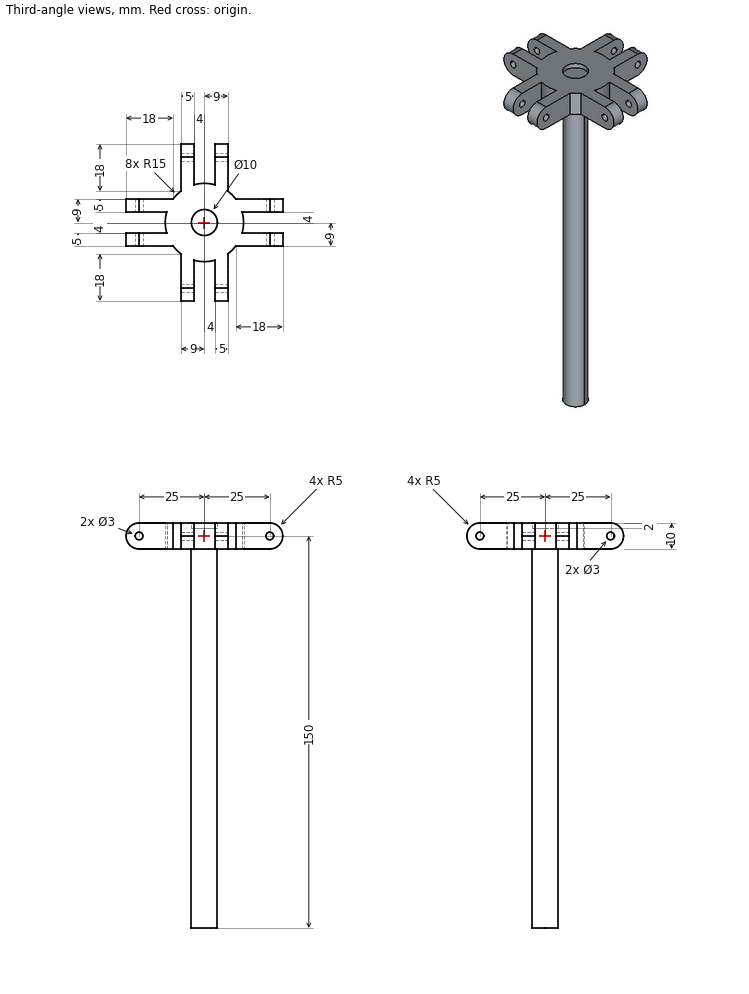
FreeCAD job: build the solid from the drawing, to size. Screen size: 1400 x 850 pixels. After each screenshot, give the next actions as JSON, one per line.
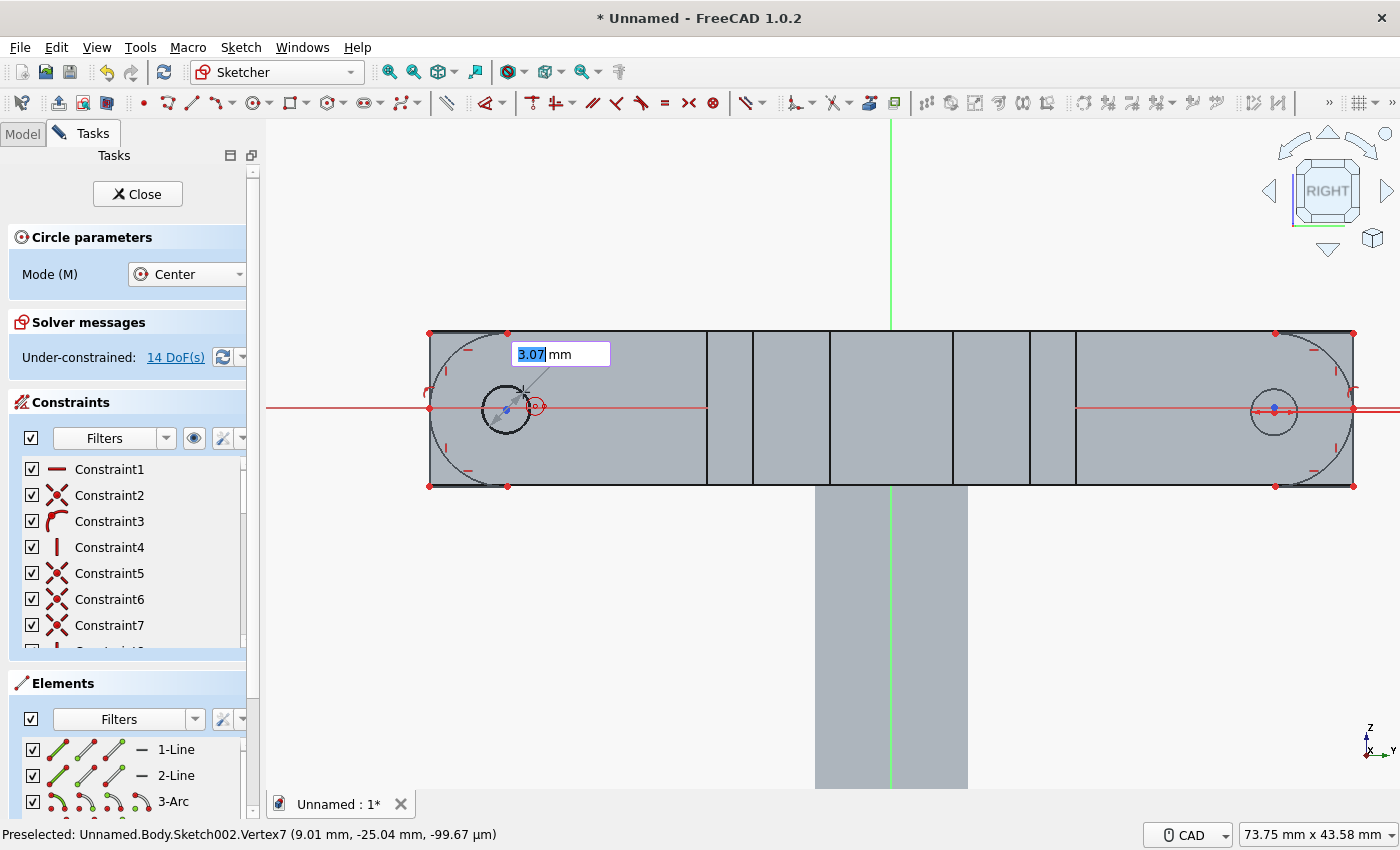
{"action": "type", "text": "3"}
{"action": "key", "text": "Return"}
{"action": "key", "text": "Escape"}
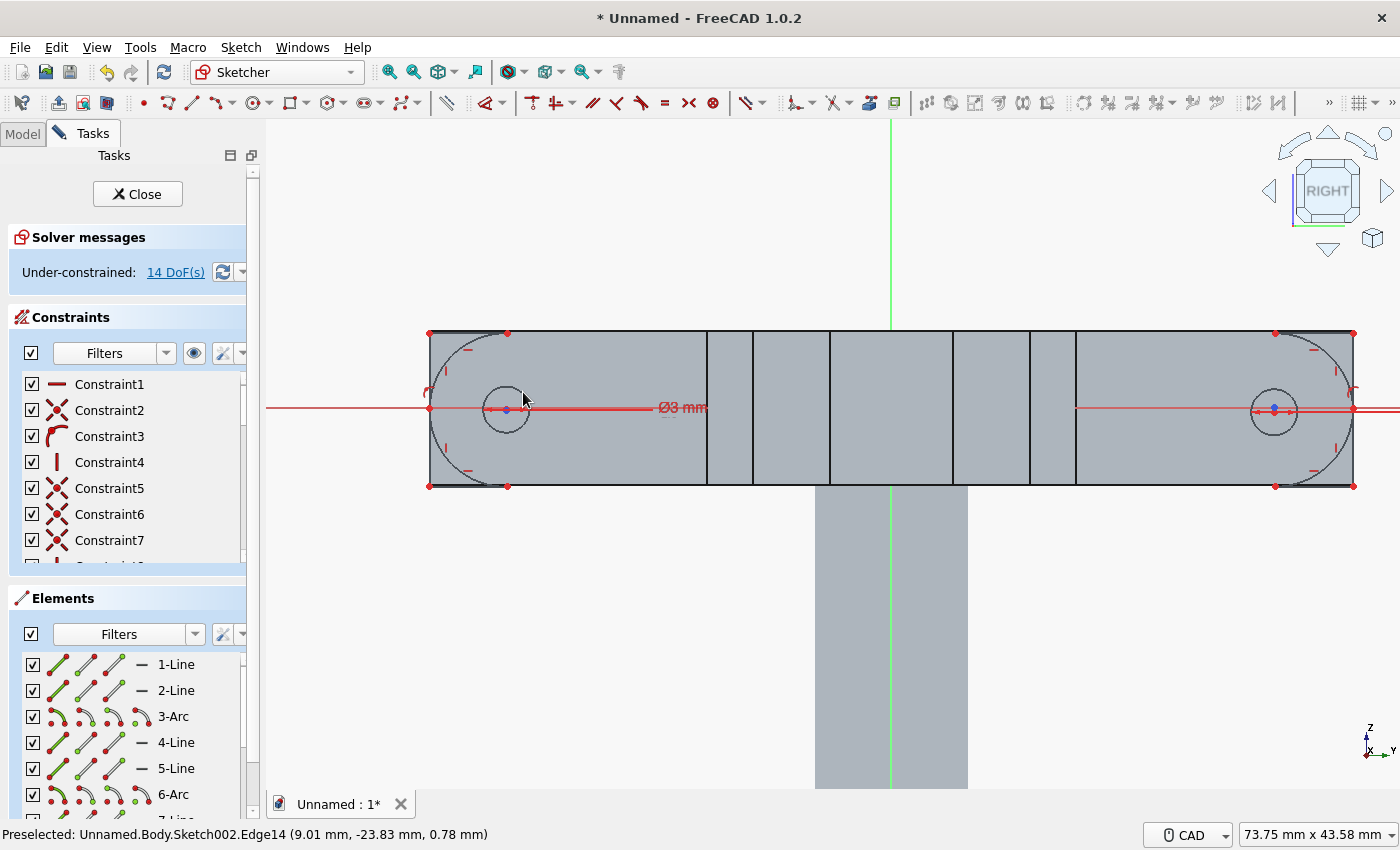
{"action": "left_click", "coordinate": [453, 333]}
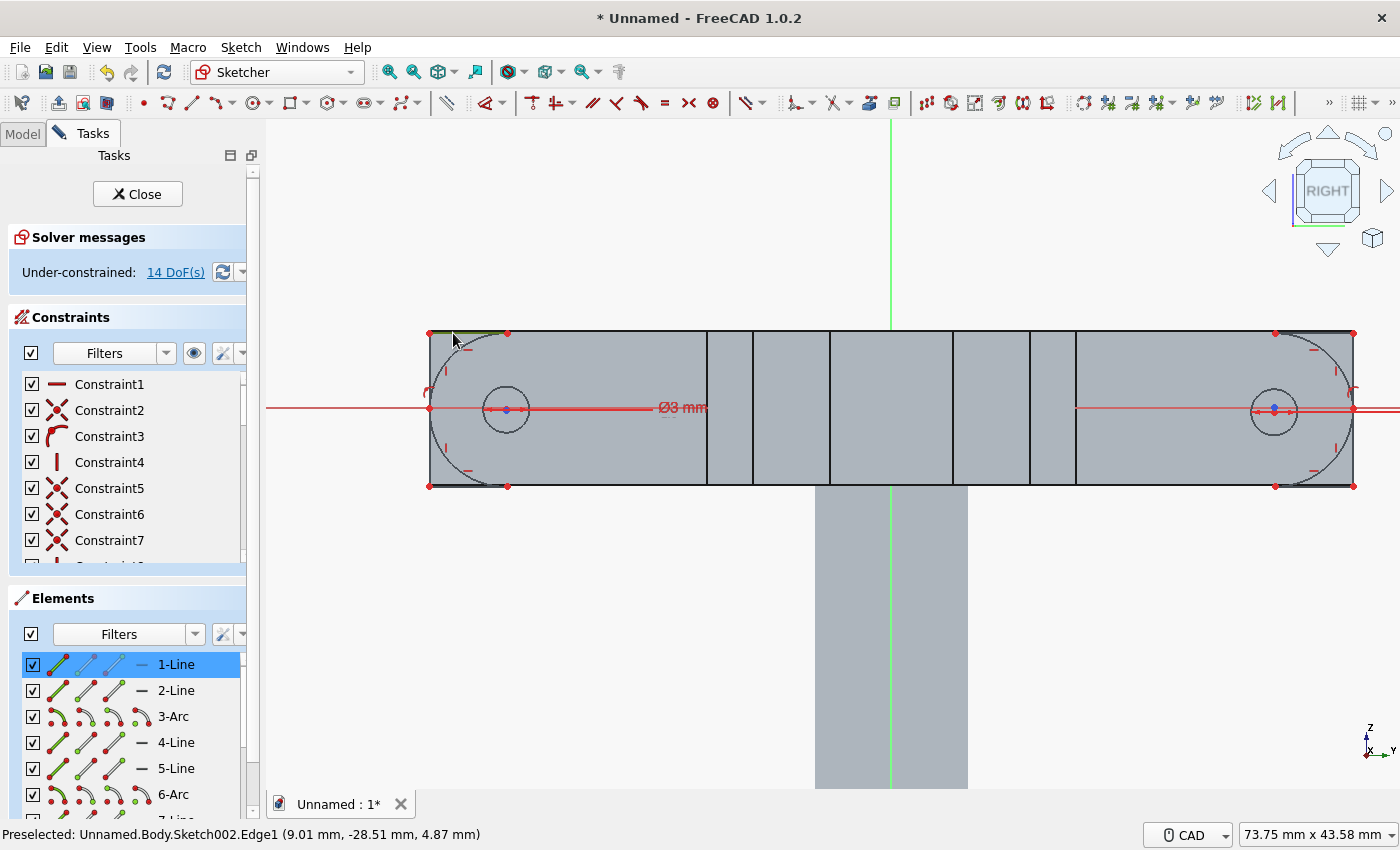
{"action": "left_click", "coordinate": [453, 355]}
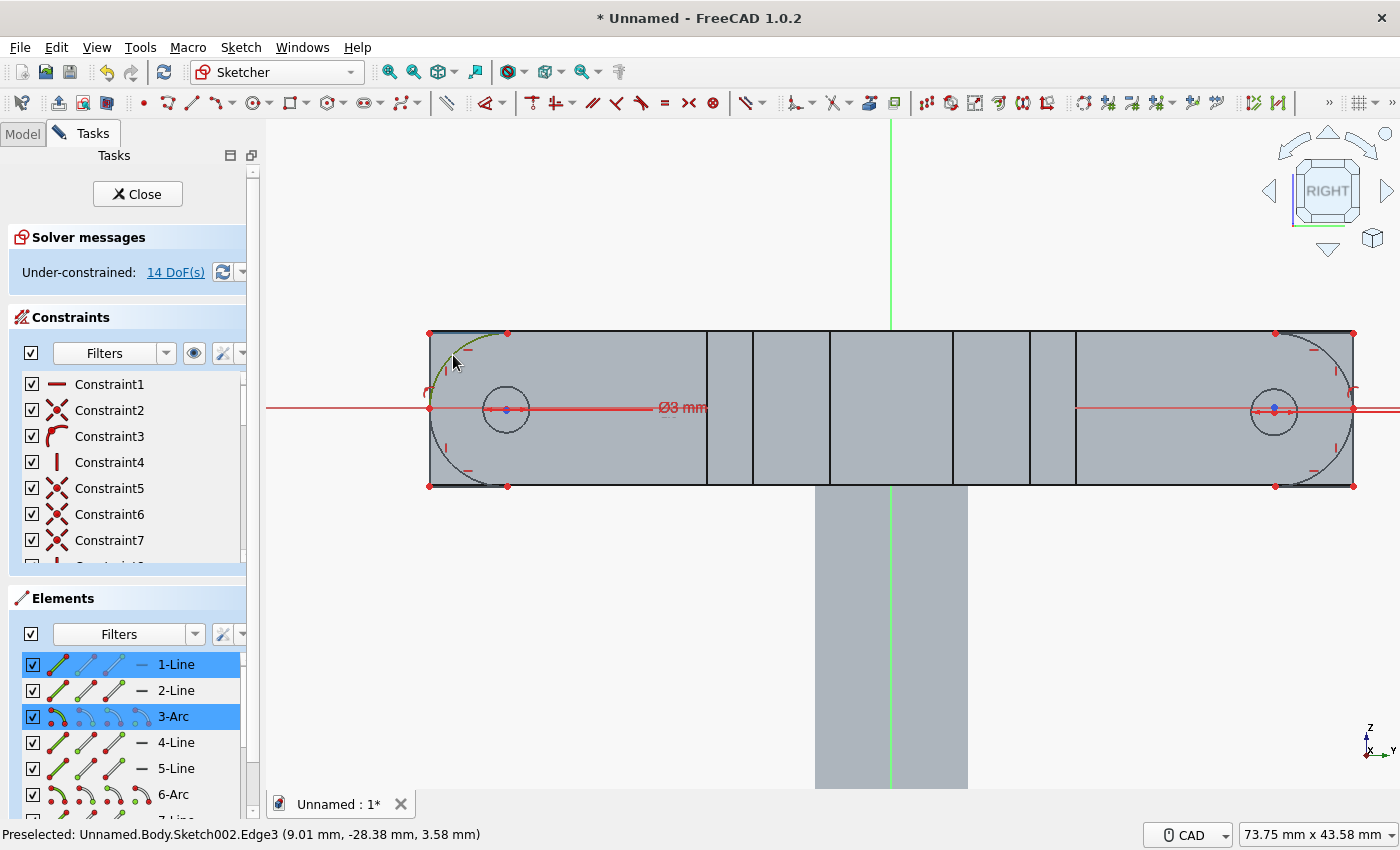
{"action": "key", "text": "t"}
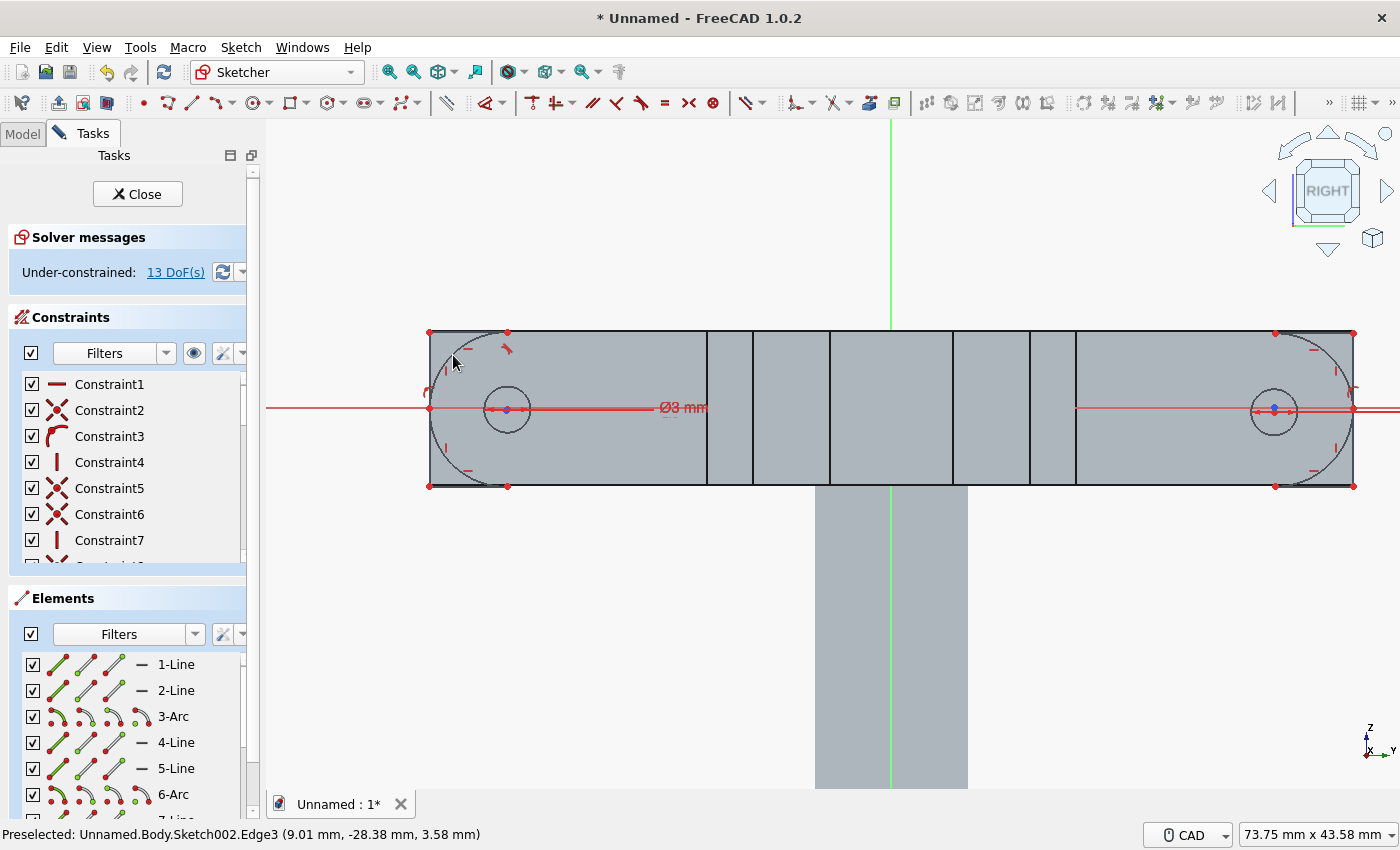
{"action": "left_click", "coordinate": [430, 355]}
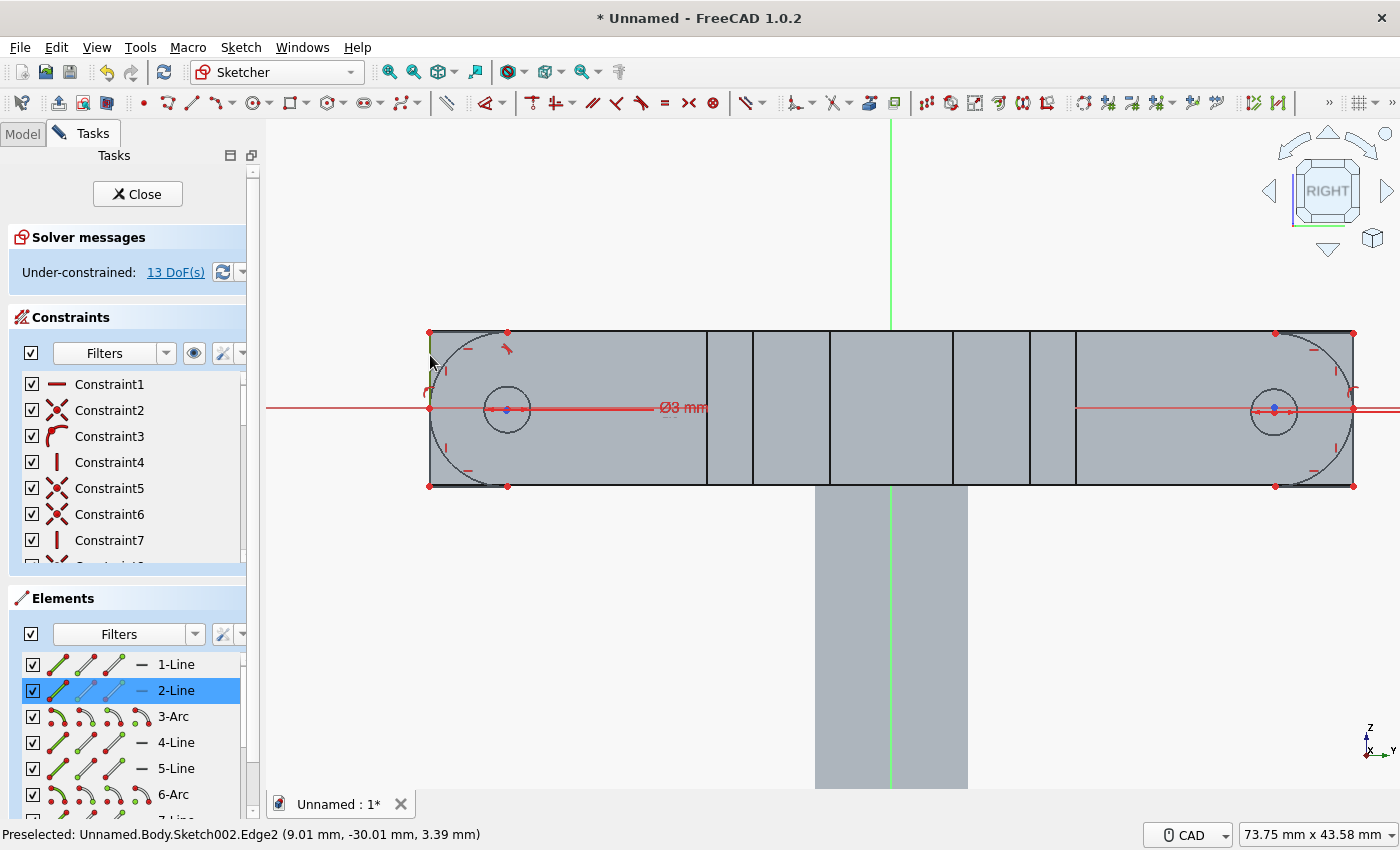
{"action": "left_click", "coordinate": [453, 354]}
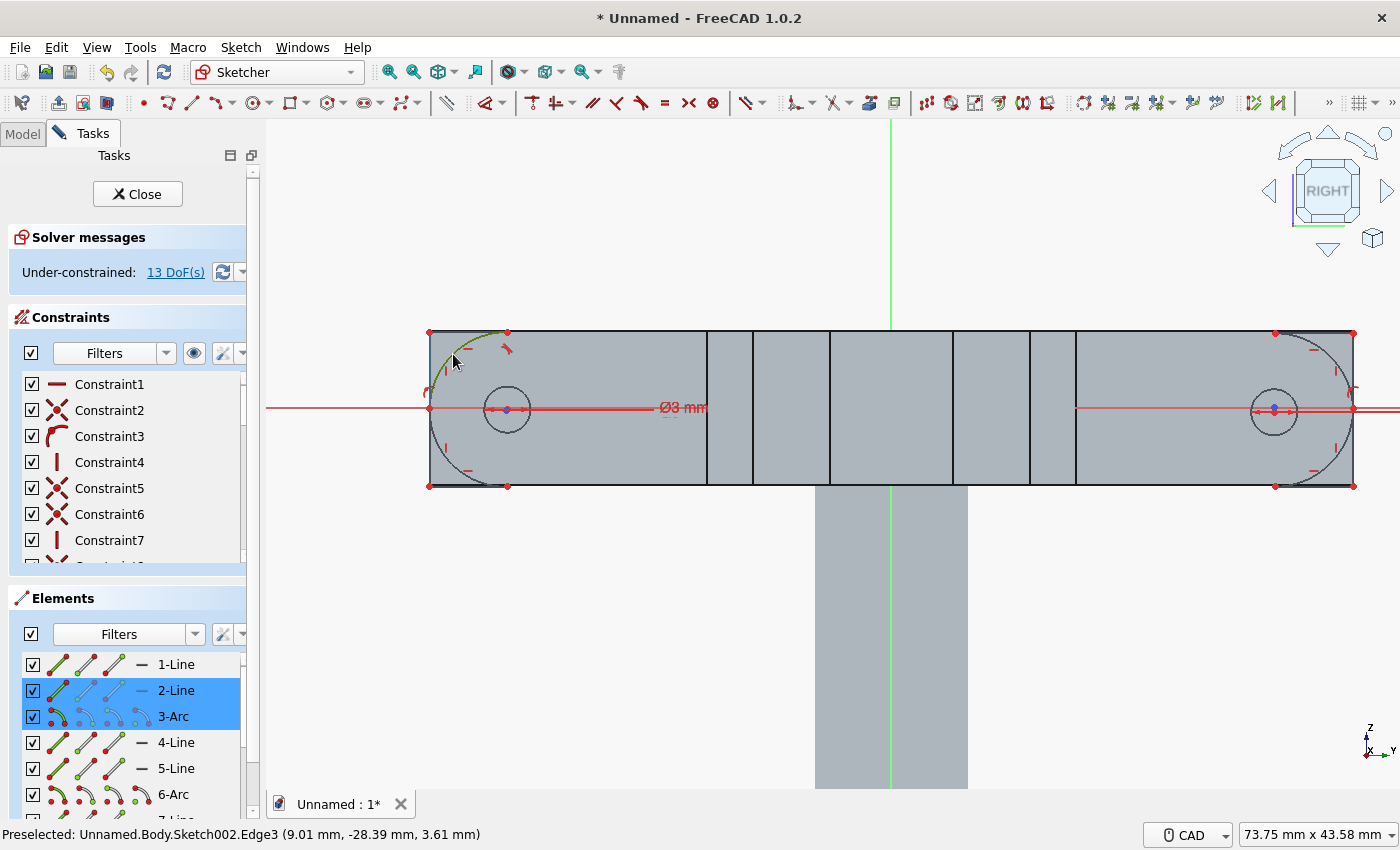
{"action": "key", "text": "t"}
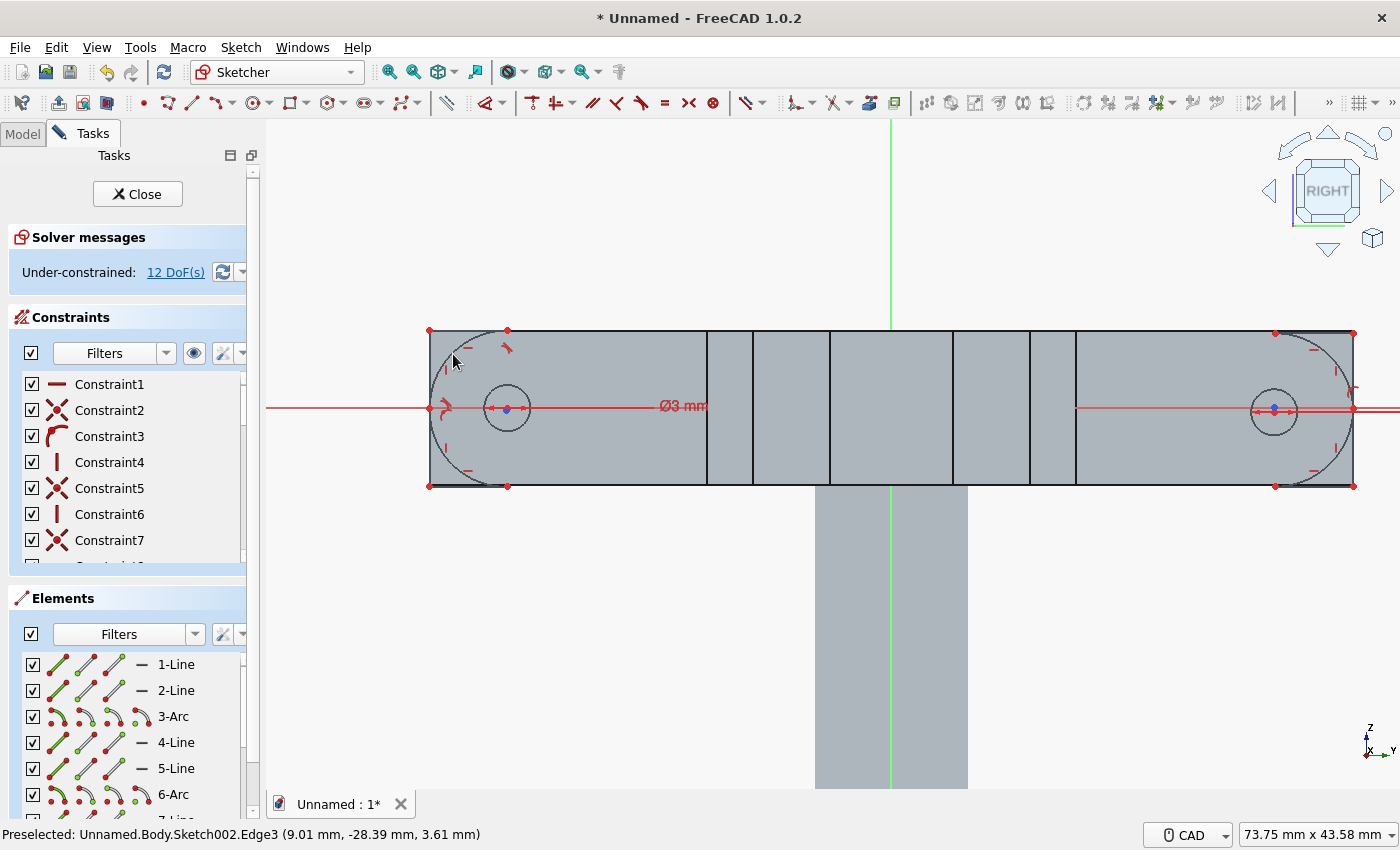
{"action": "left_click", "coordinate": [430, 354]}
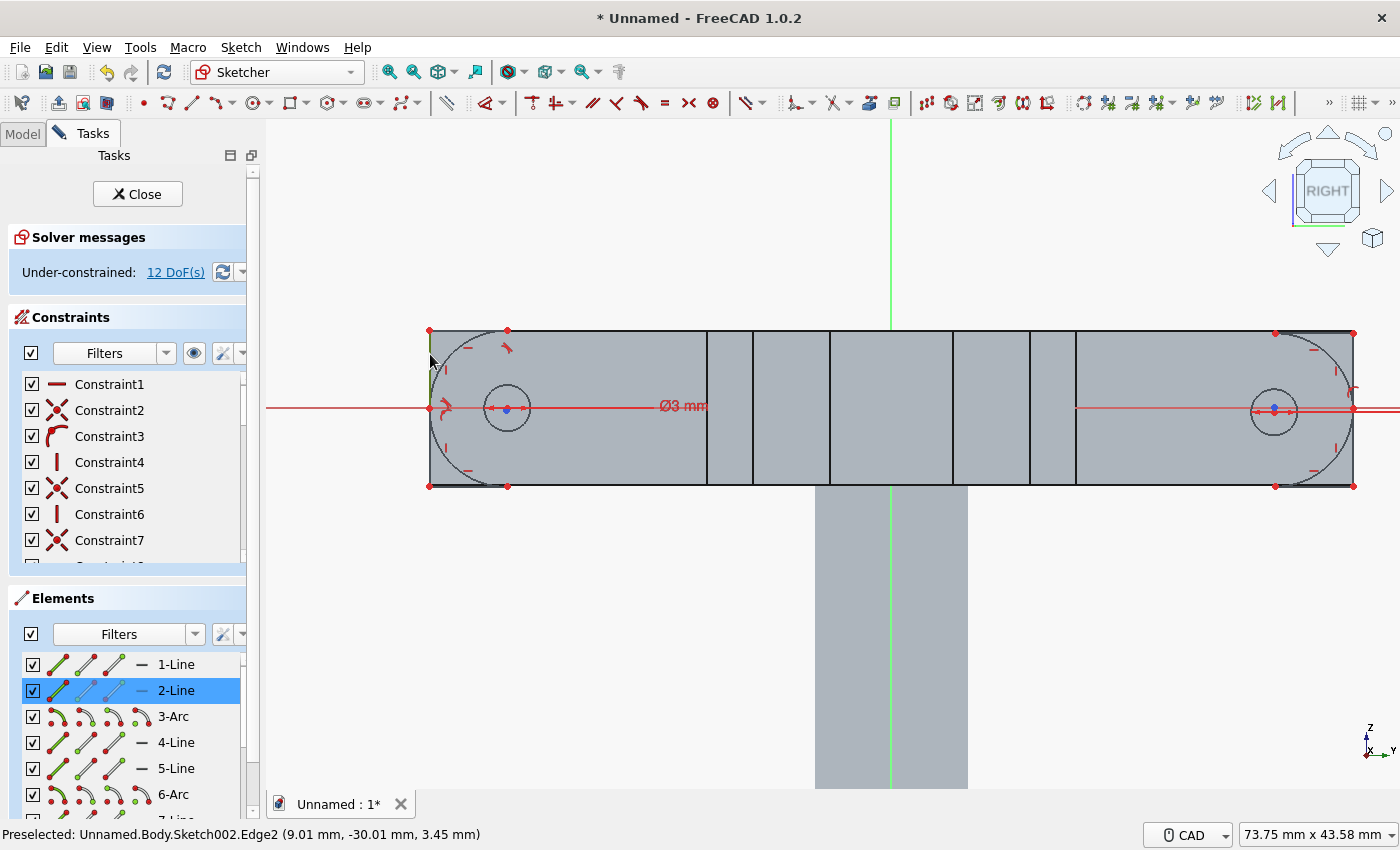
{"action": "left_click", "coordinate": [452, 464]}